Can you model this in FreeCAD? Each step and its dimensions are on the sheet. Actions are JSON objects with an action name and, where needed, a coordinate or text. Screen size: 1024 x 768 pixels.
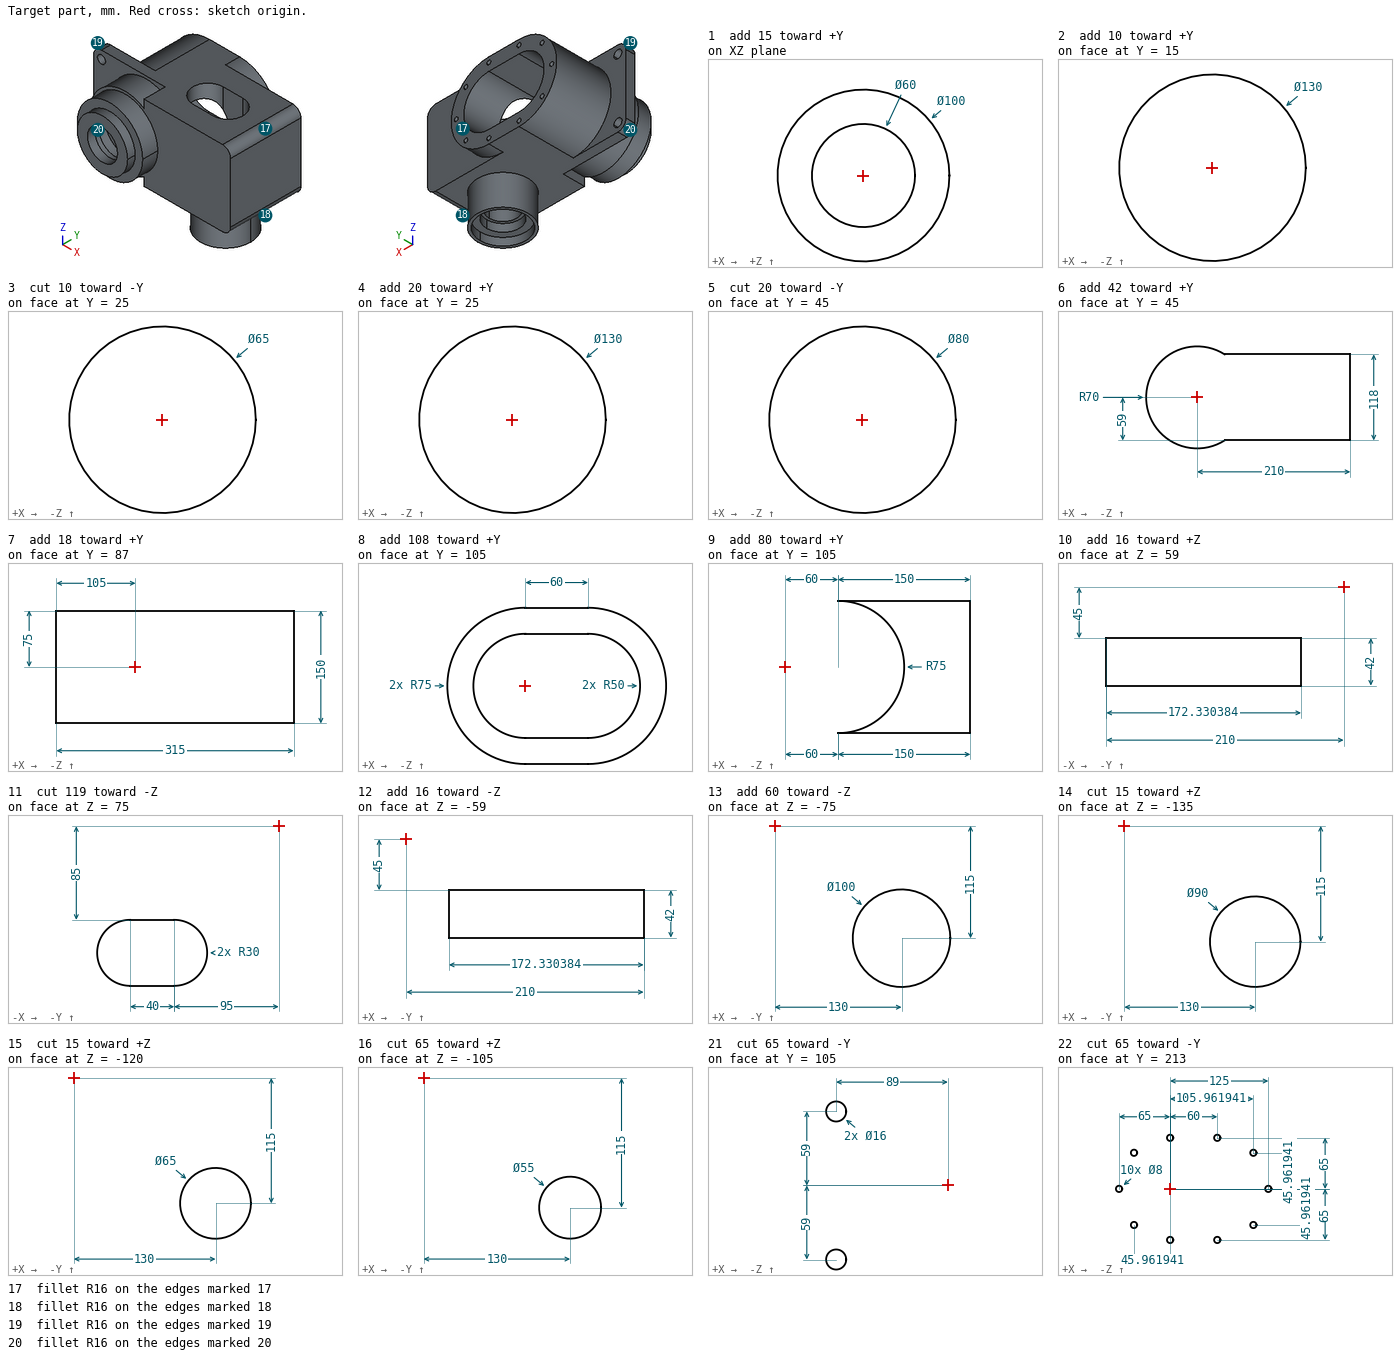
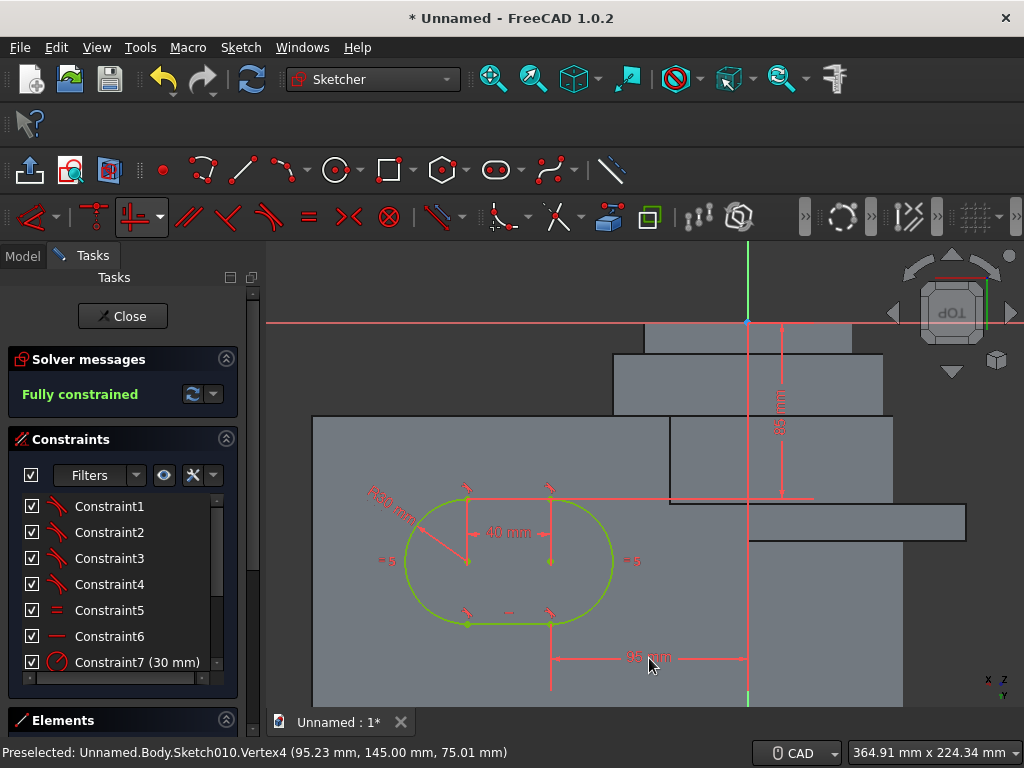
{"action": "left_click", "coordinate": [123, 316]}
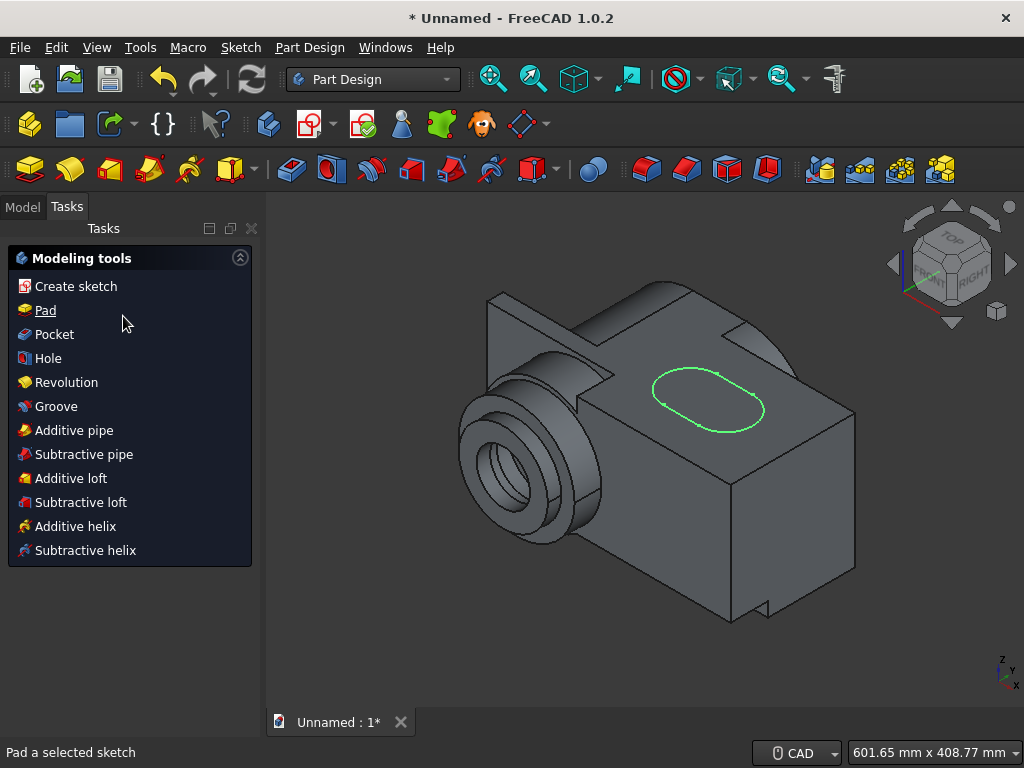
{"action": "left_click", "coordinate": [292, 170]}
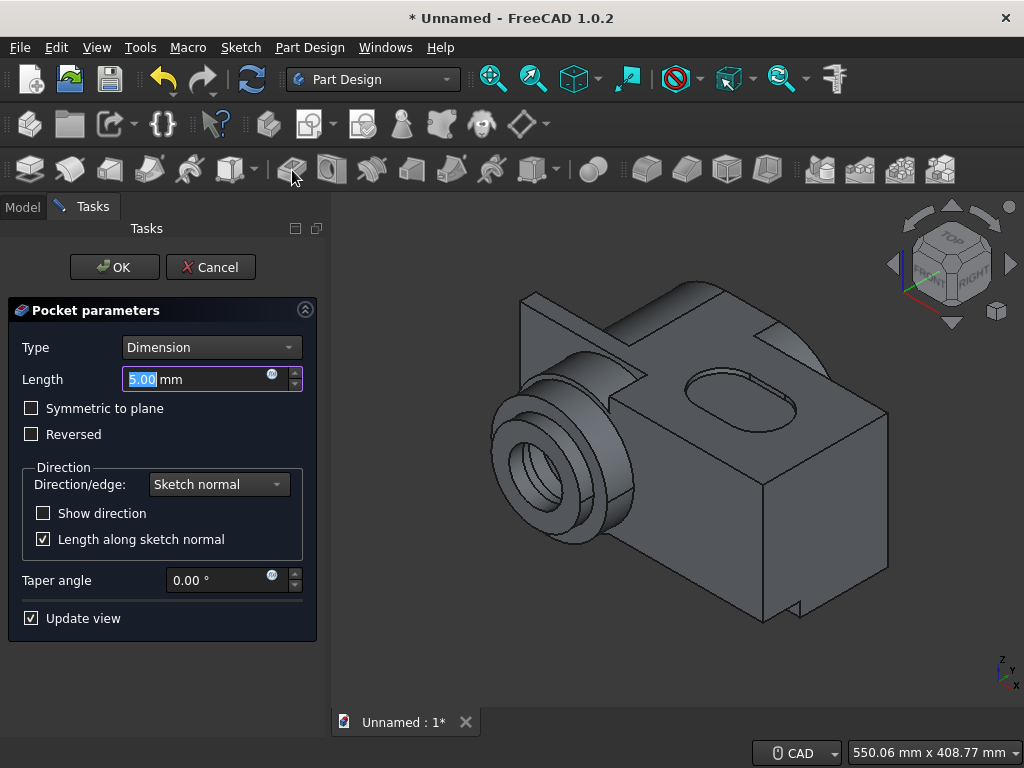
{"action": "type", "text": "119"}
{"action": "key", "text": "Tab"}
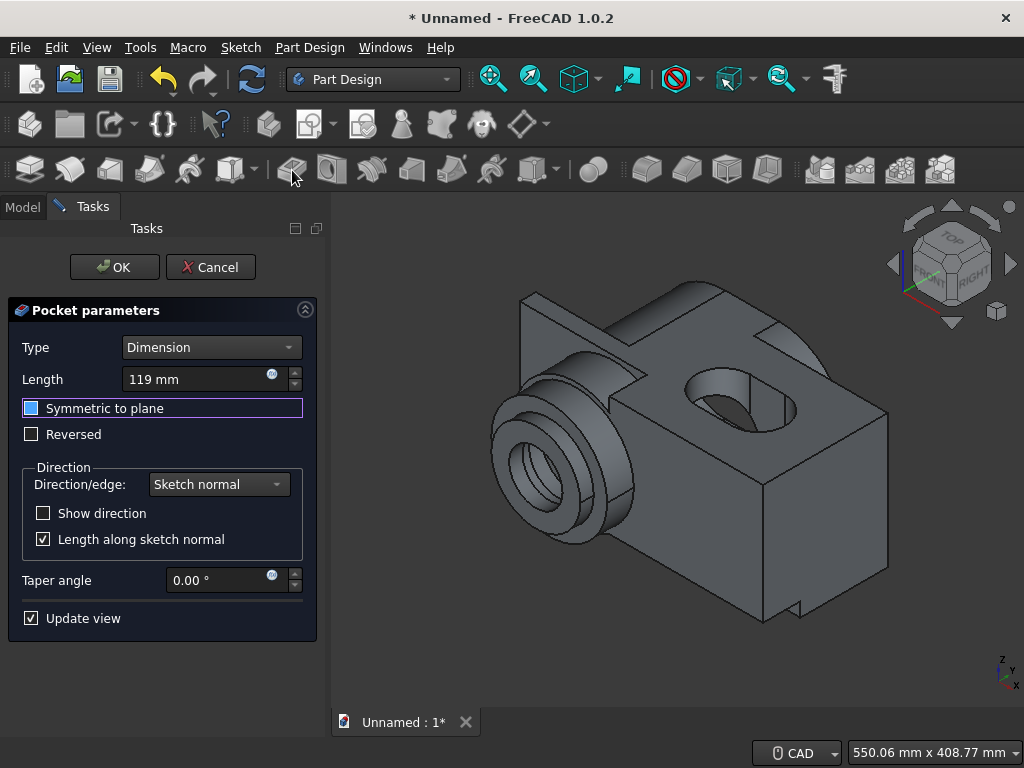
{"action": "left_click", "coordinate": [115, 267]}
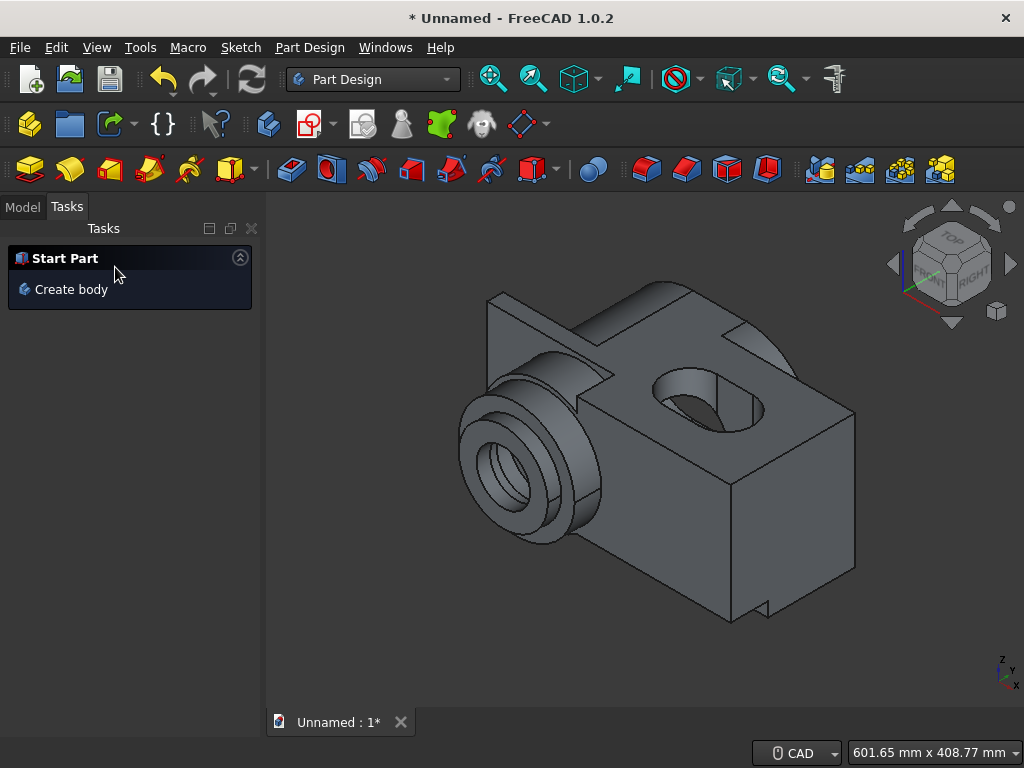
{"action": "key", "text": "5"}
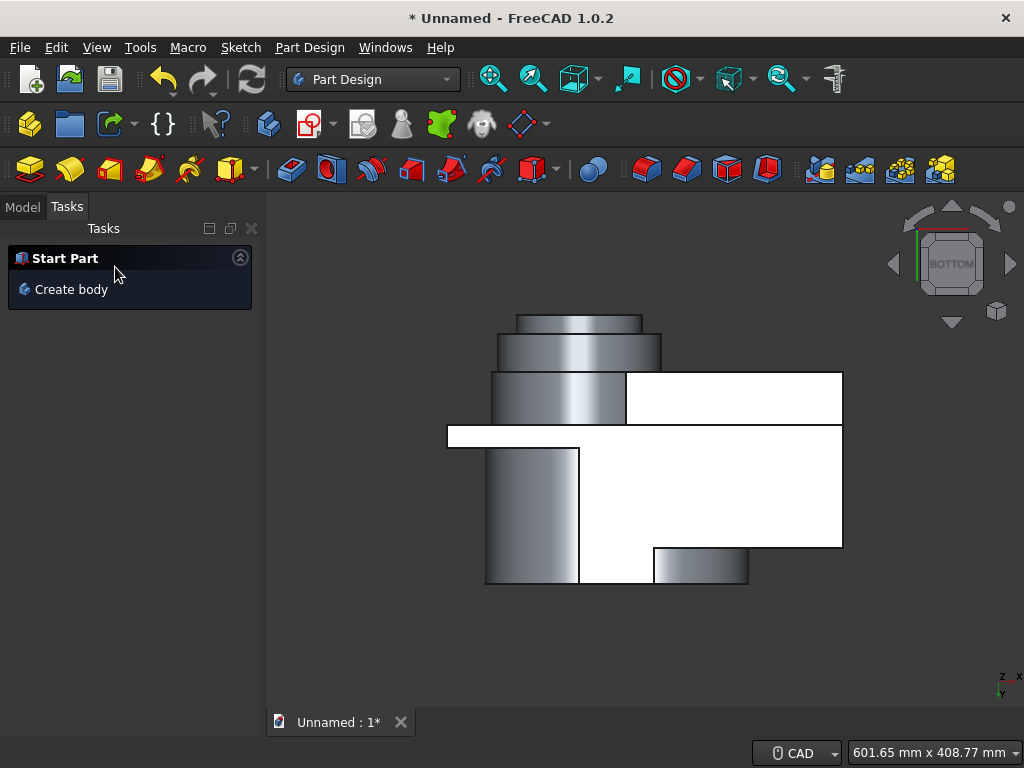
{"action": "left_click", "coordinate": [797, 397]}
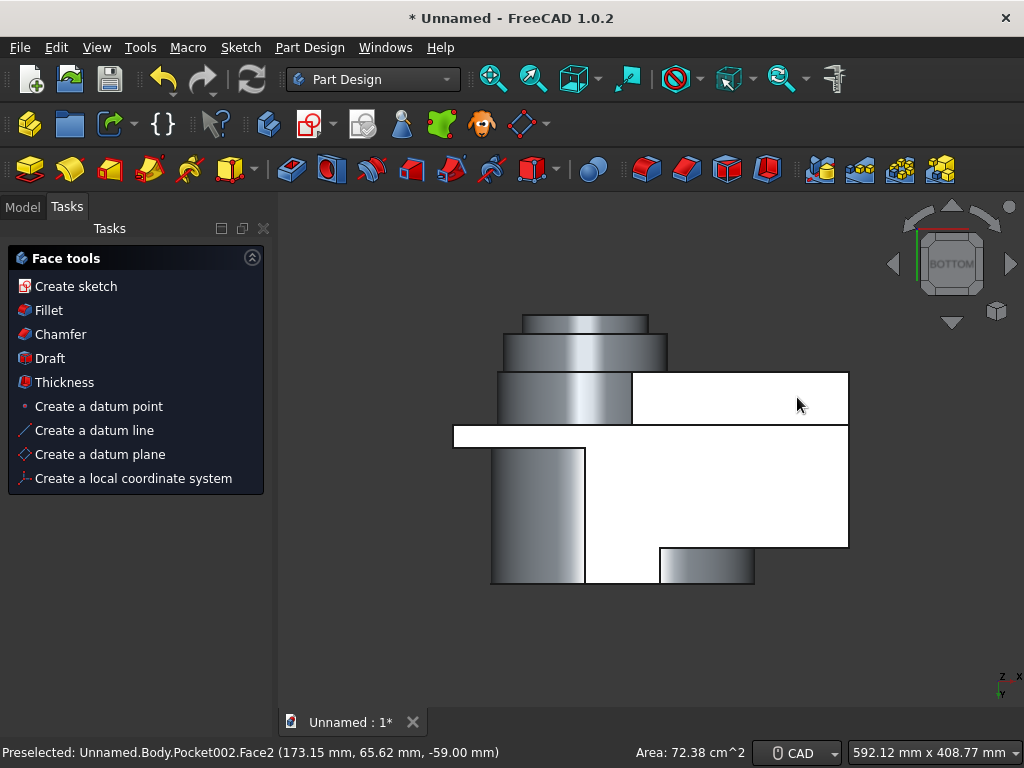
{"action": "left_click", "coordinate": [310, 124]}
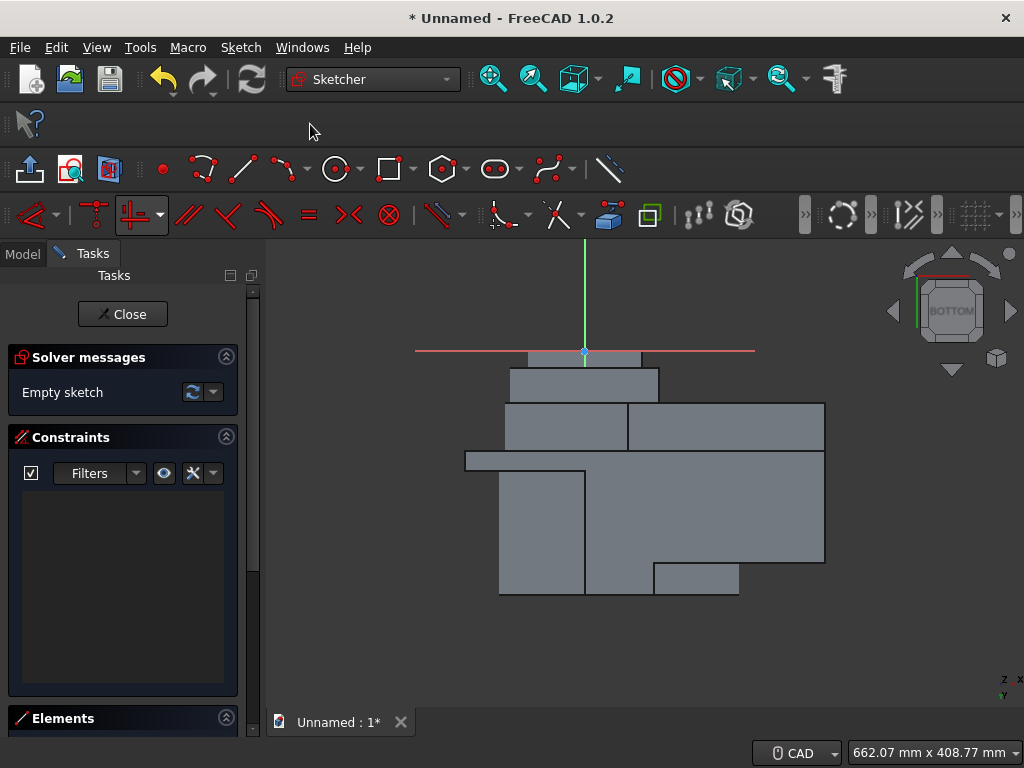
{"action": "scroll", "coordinate": [859, 313], "scroll_direction": "up", "scroll_amount": 3}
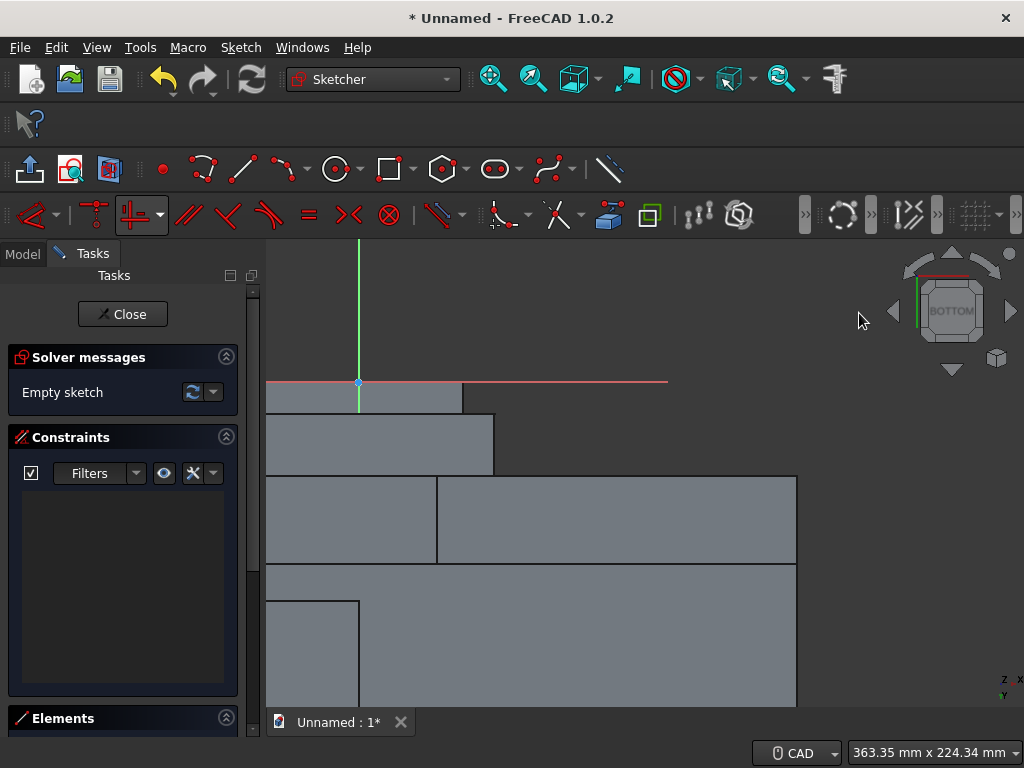
{"action": "left_click", "coordinate": [390, 170]}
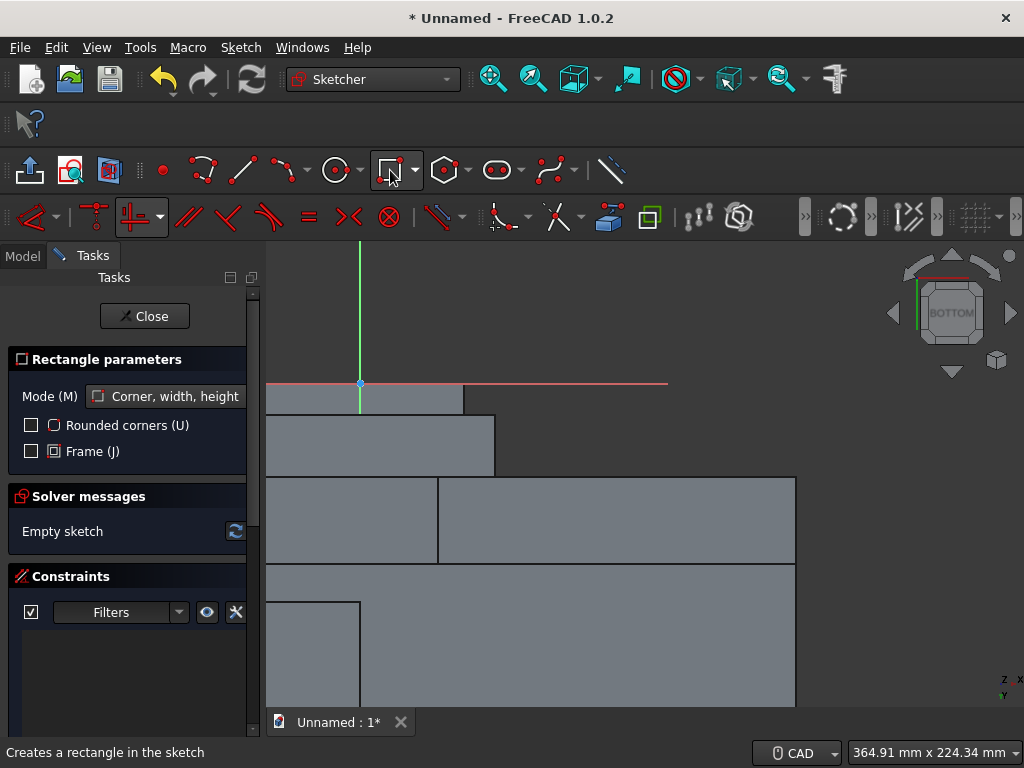
{"action": "left_click", "coordinate": [438, 477]}
{"action": "mouse_move", "coordinate": [796, 564]}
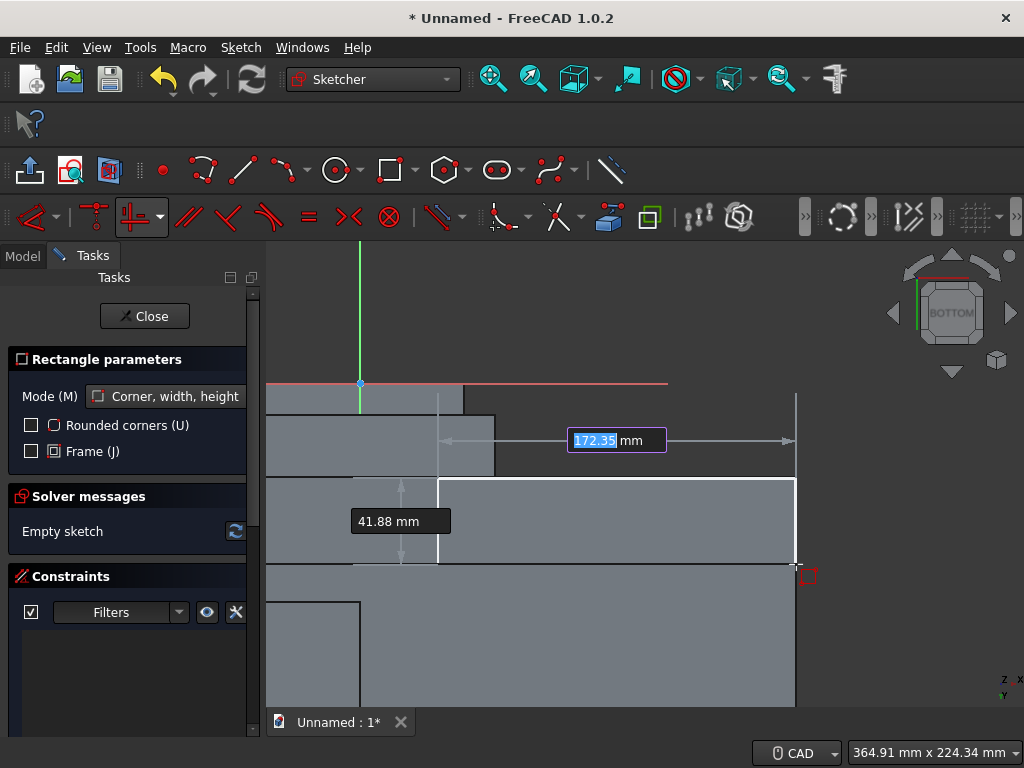
{"action": "type", "text": "172.330384"}
{"action": "key", "text": "Tab"}
{"action": "type", "text": "42"}
{"action": "key", "text": "Return"}
{"action": "key", "text": "Escape"}